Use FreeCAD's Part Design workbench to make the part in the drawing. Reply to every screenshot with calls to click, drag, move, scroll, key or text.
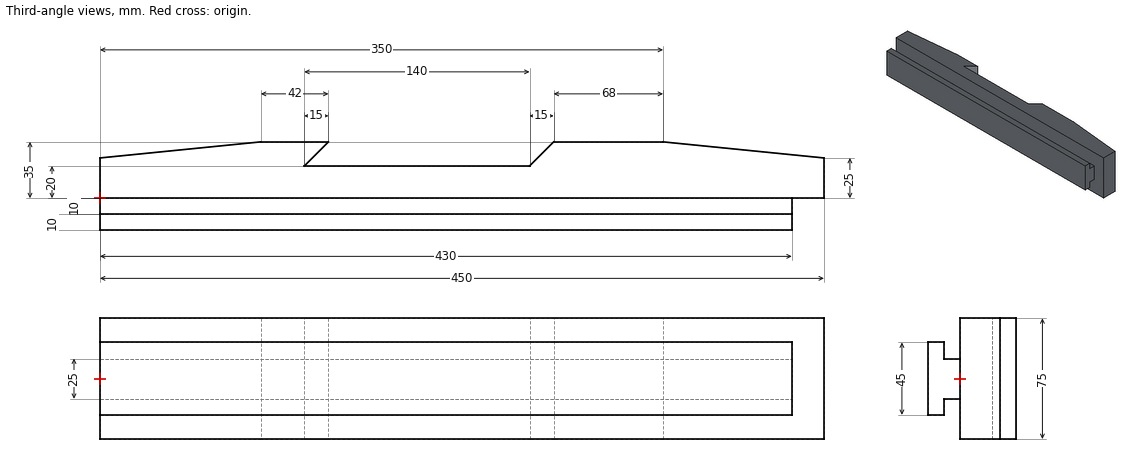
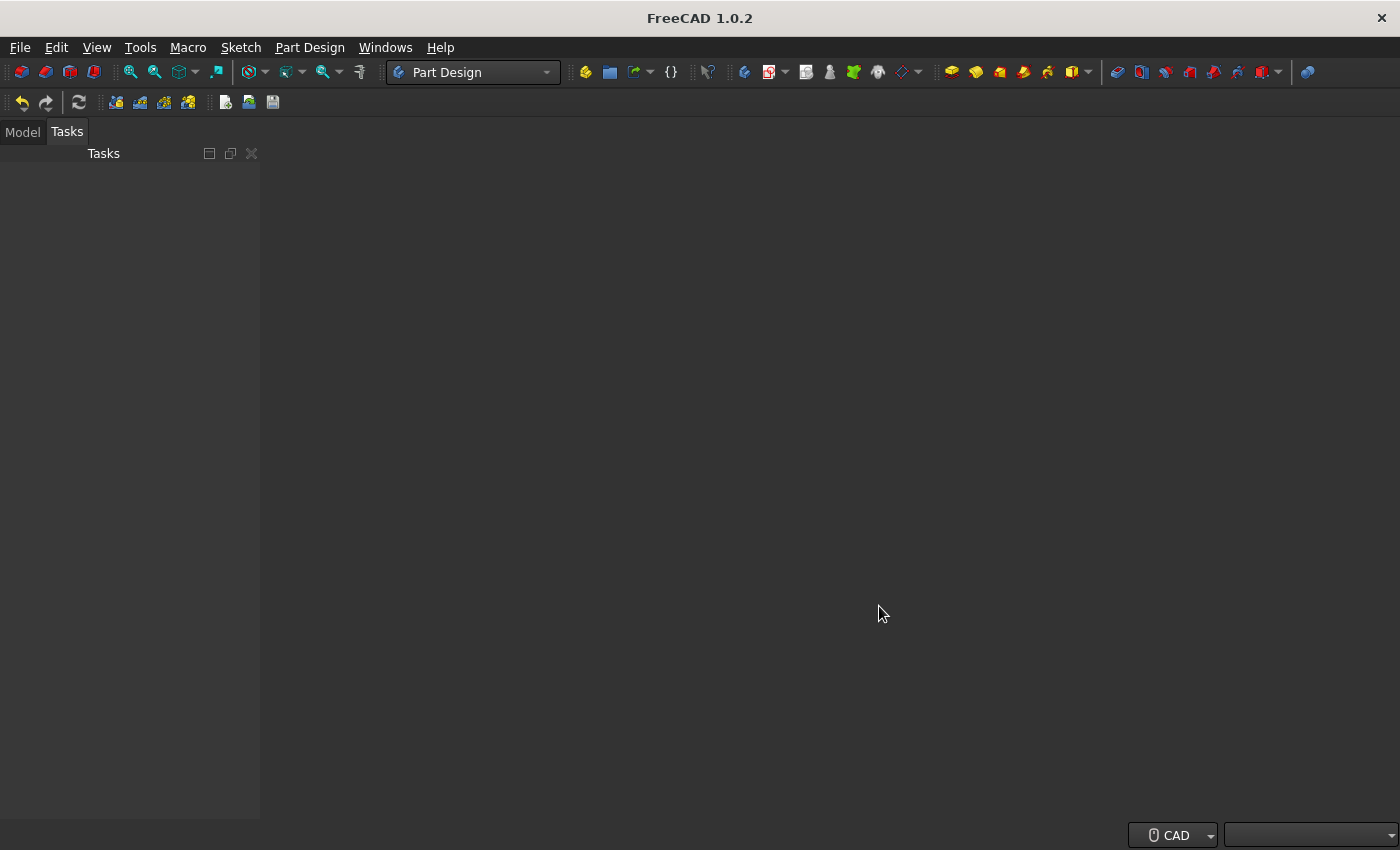
click(226, 102)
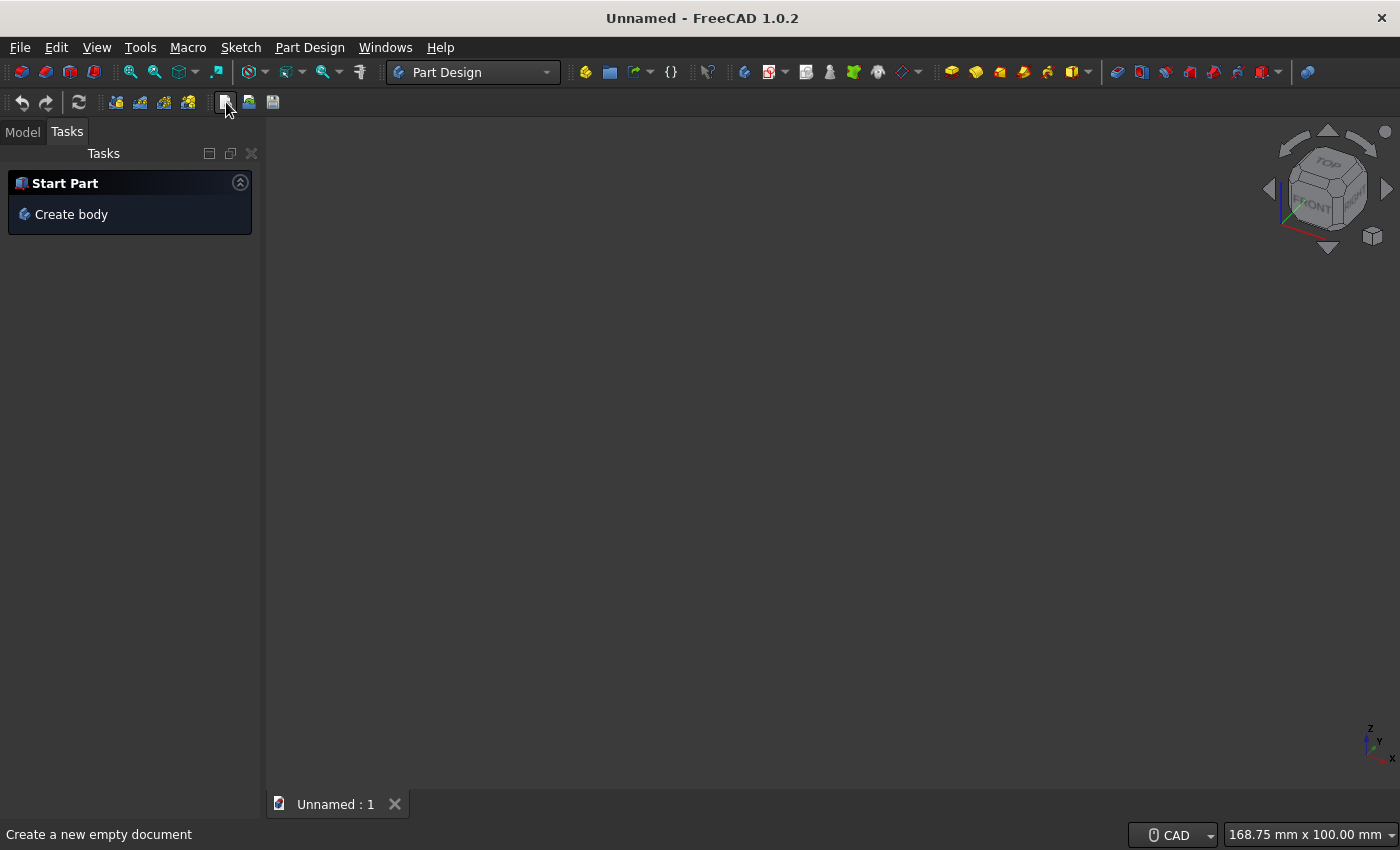
click(770, 72)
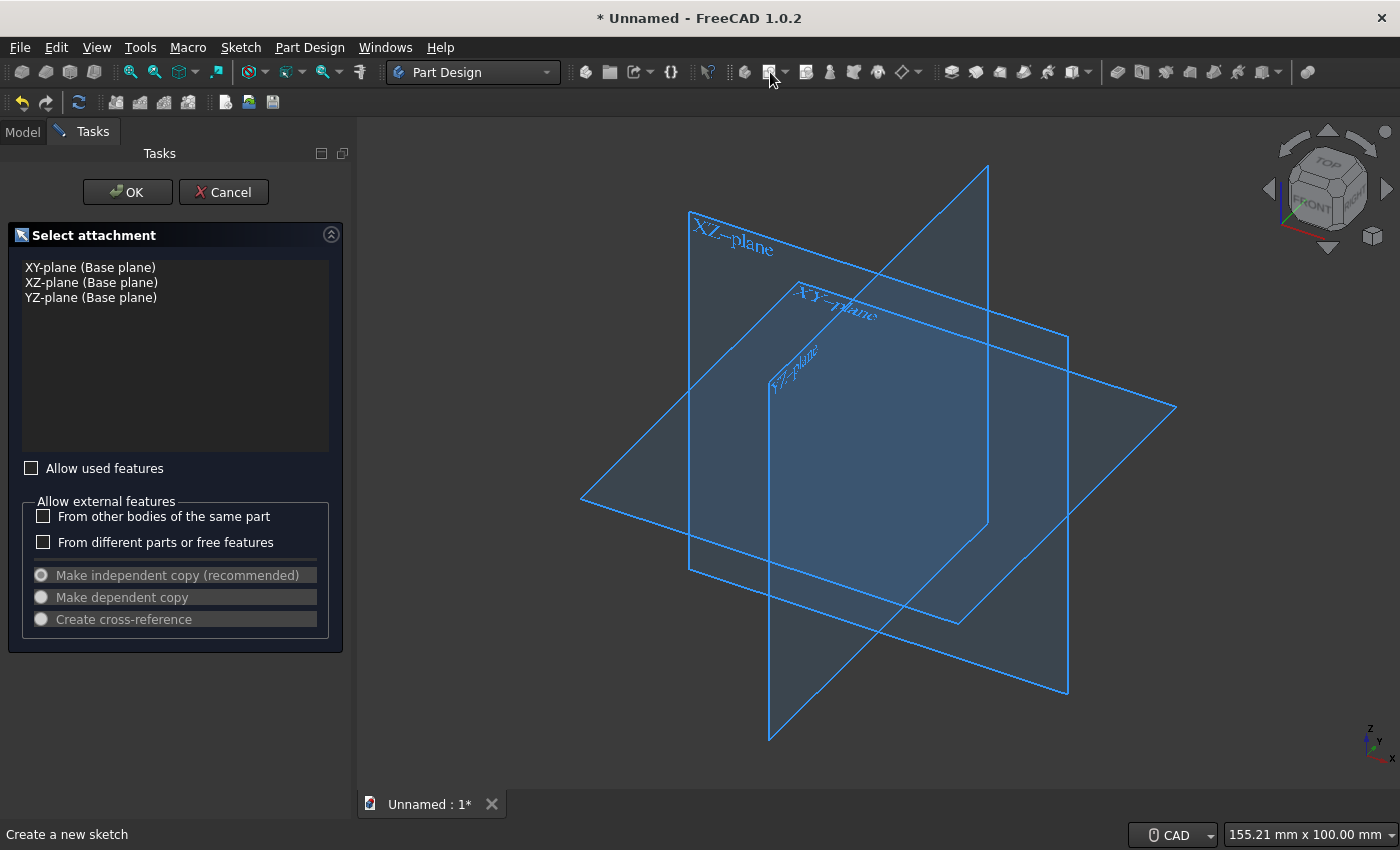
click(82, 268)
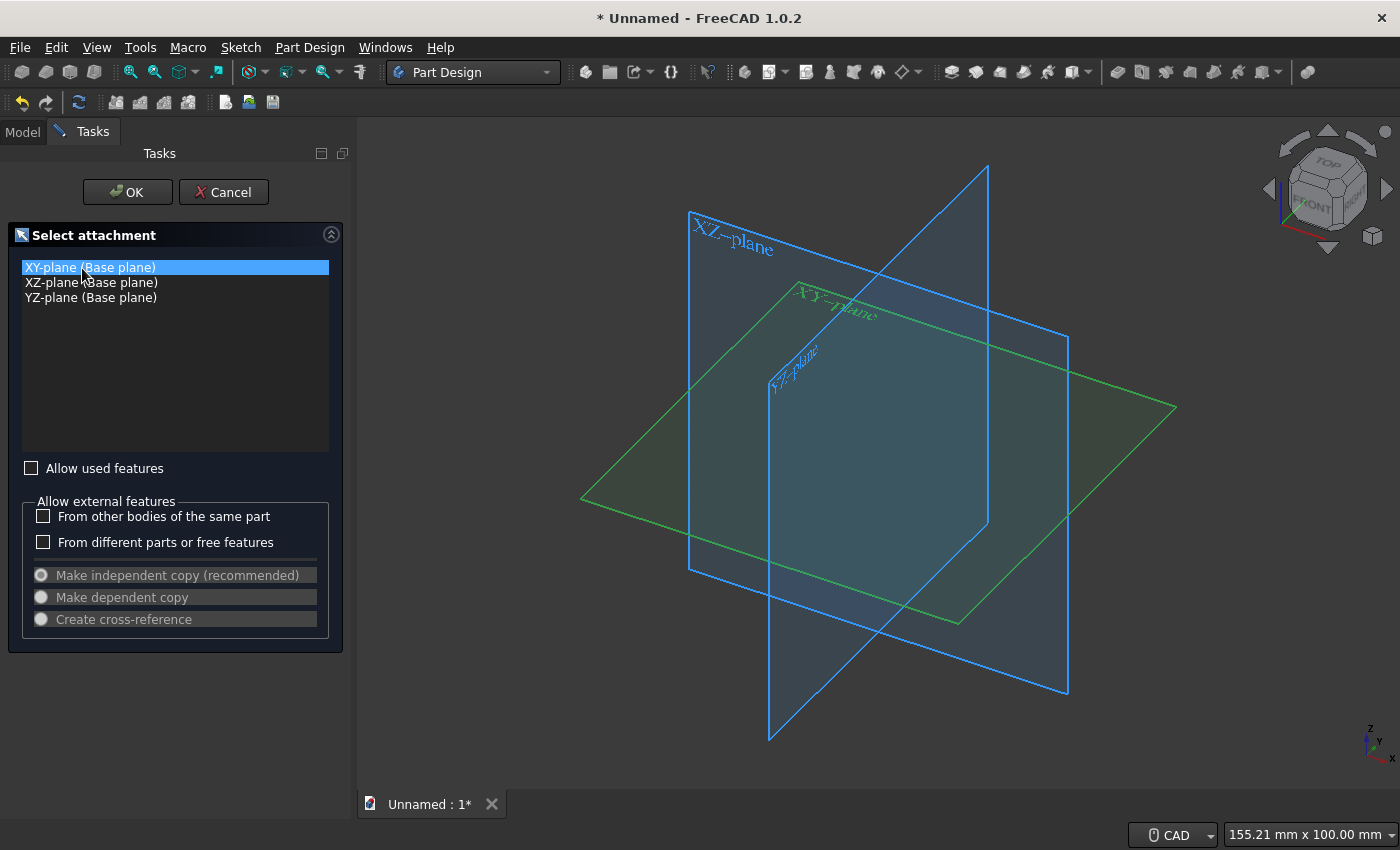
click(128, 192)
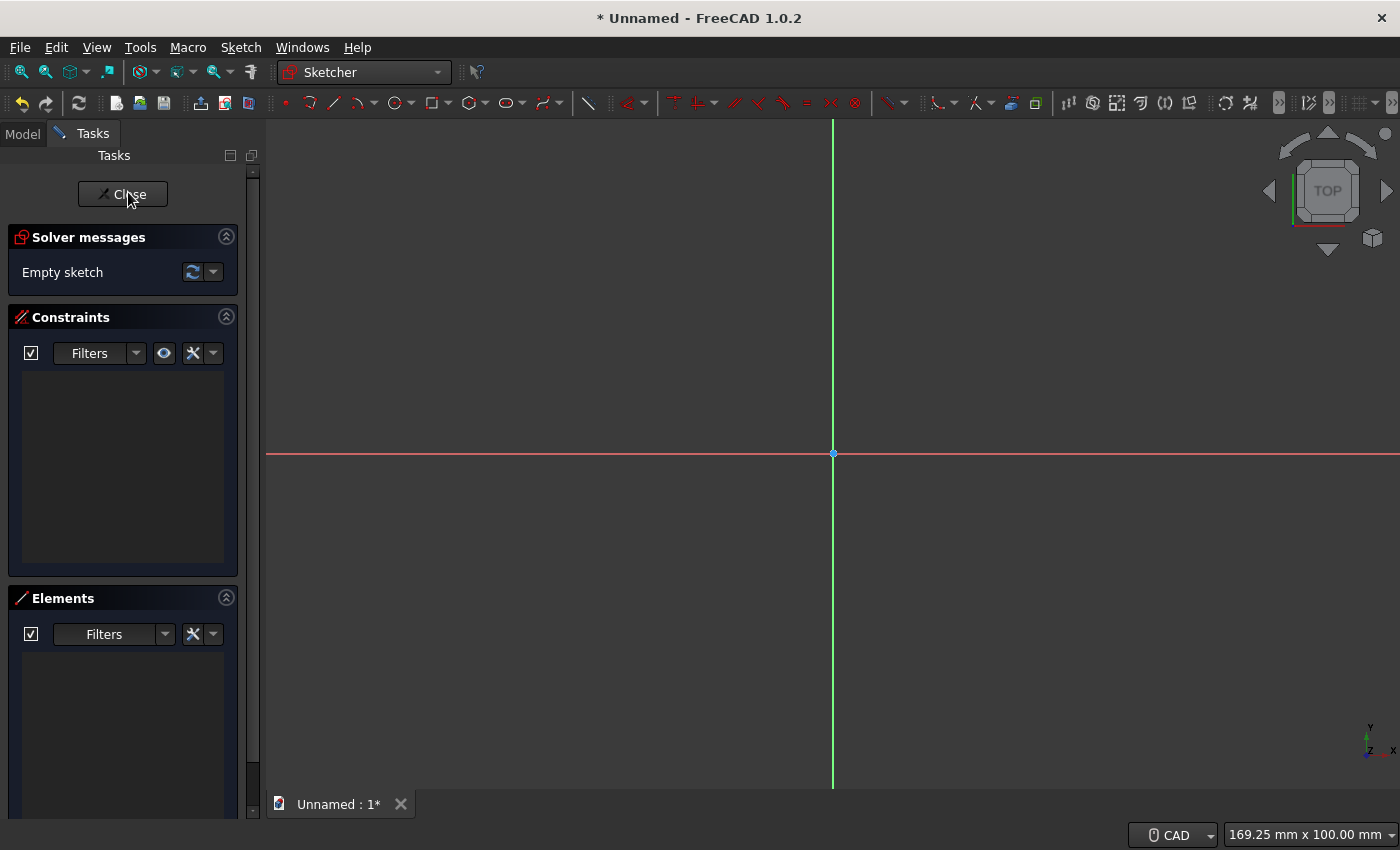
scroll(366, 484, down, 8)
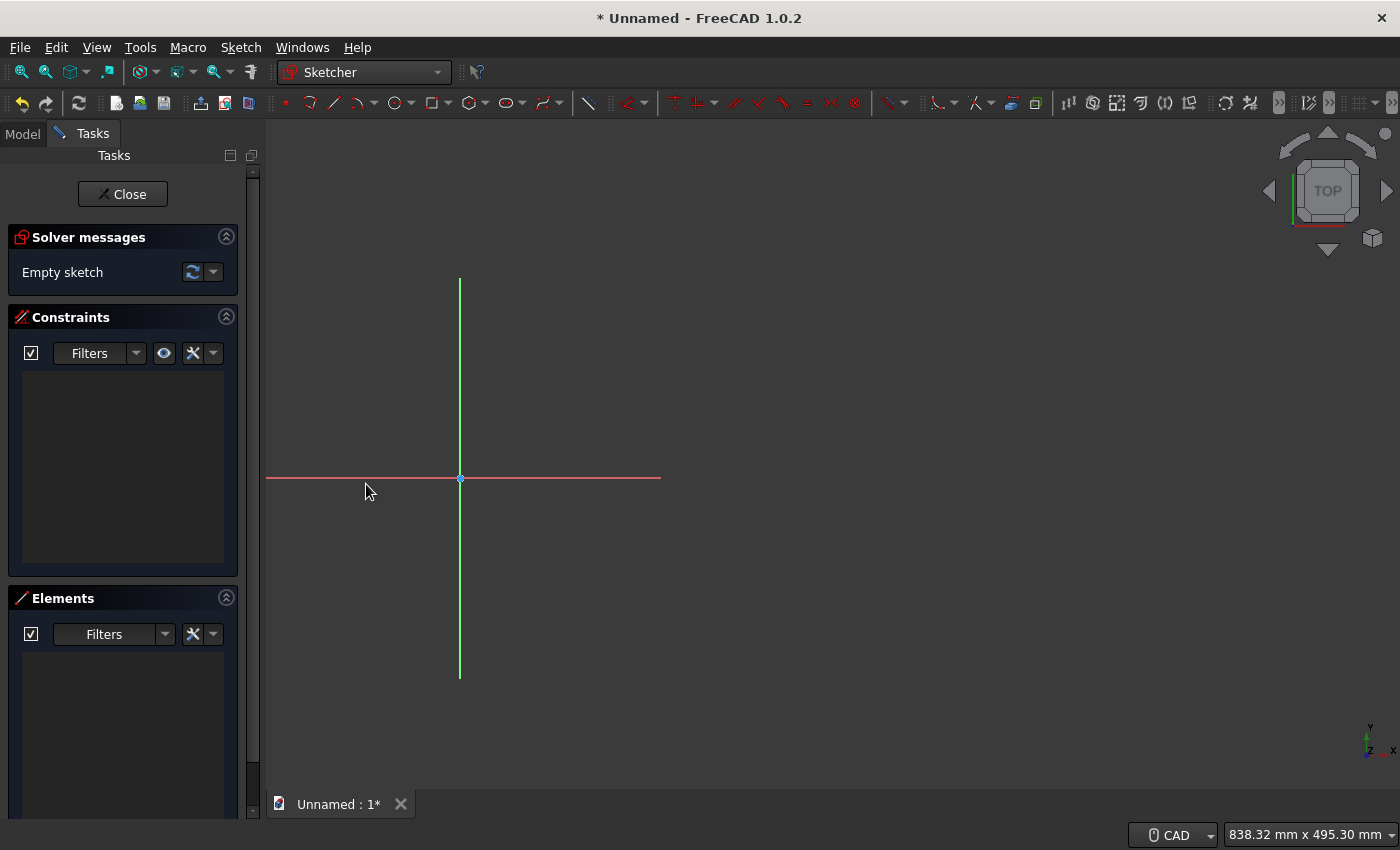
click(310, 104)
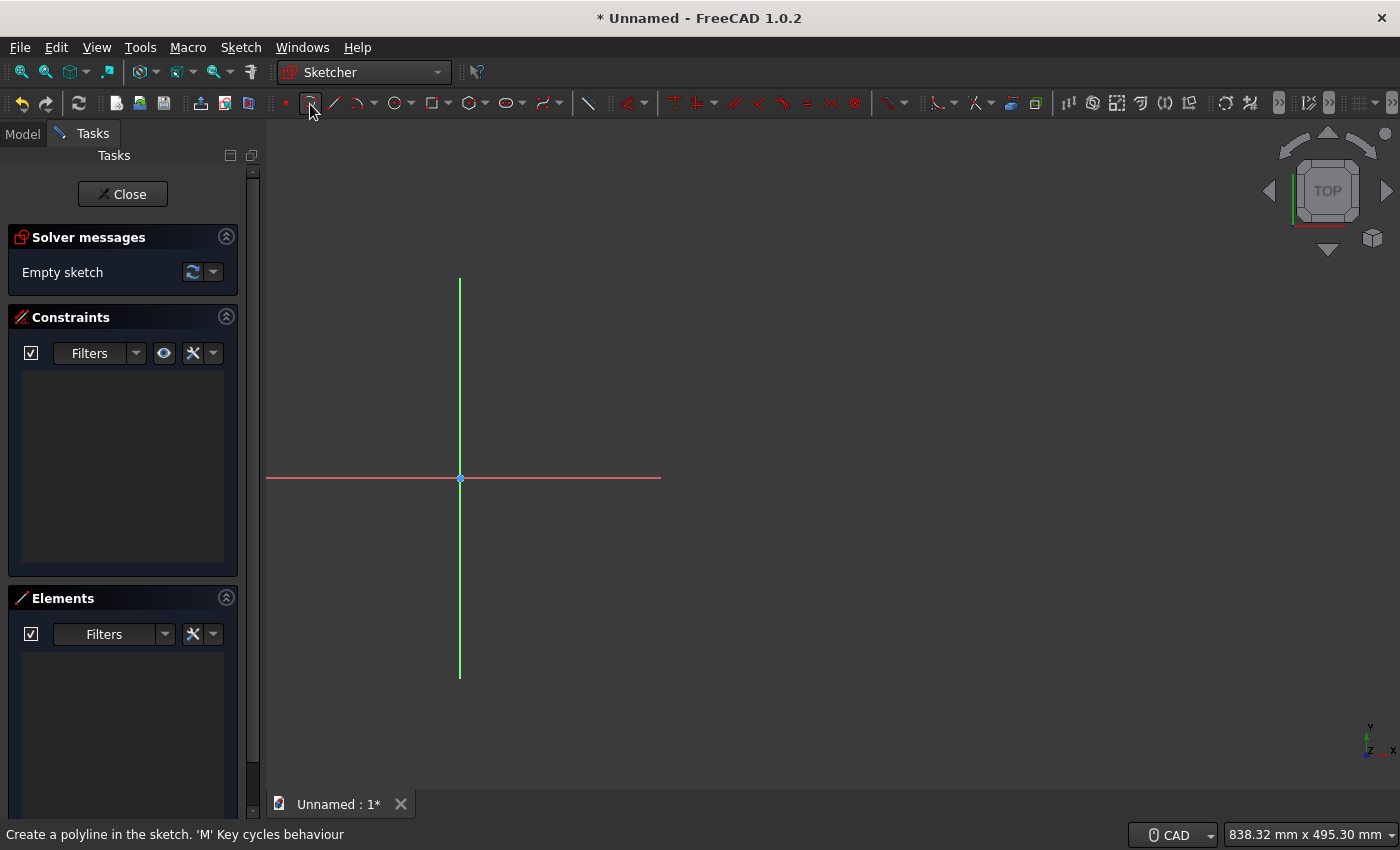
click(460, 478)
click(1069, 469)
click(1069, 445)
click(934, 431)
click(842, 431)
click(822, 451)
click(632, 451)
click(652, 431)
click(596, 431)
click(469, 445)
click(460, 478)
key(Escape)
key(Escape)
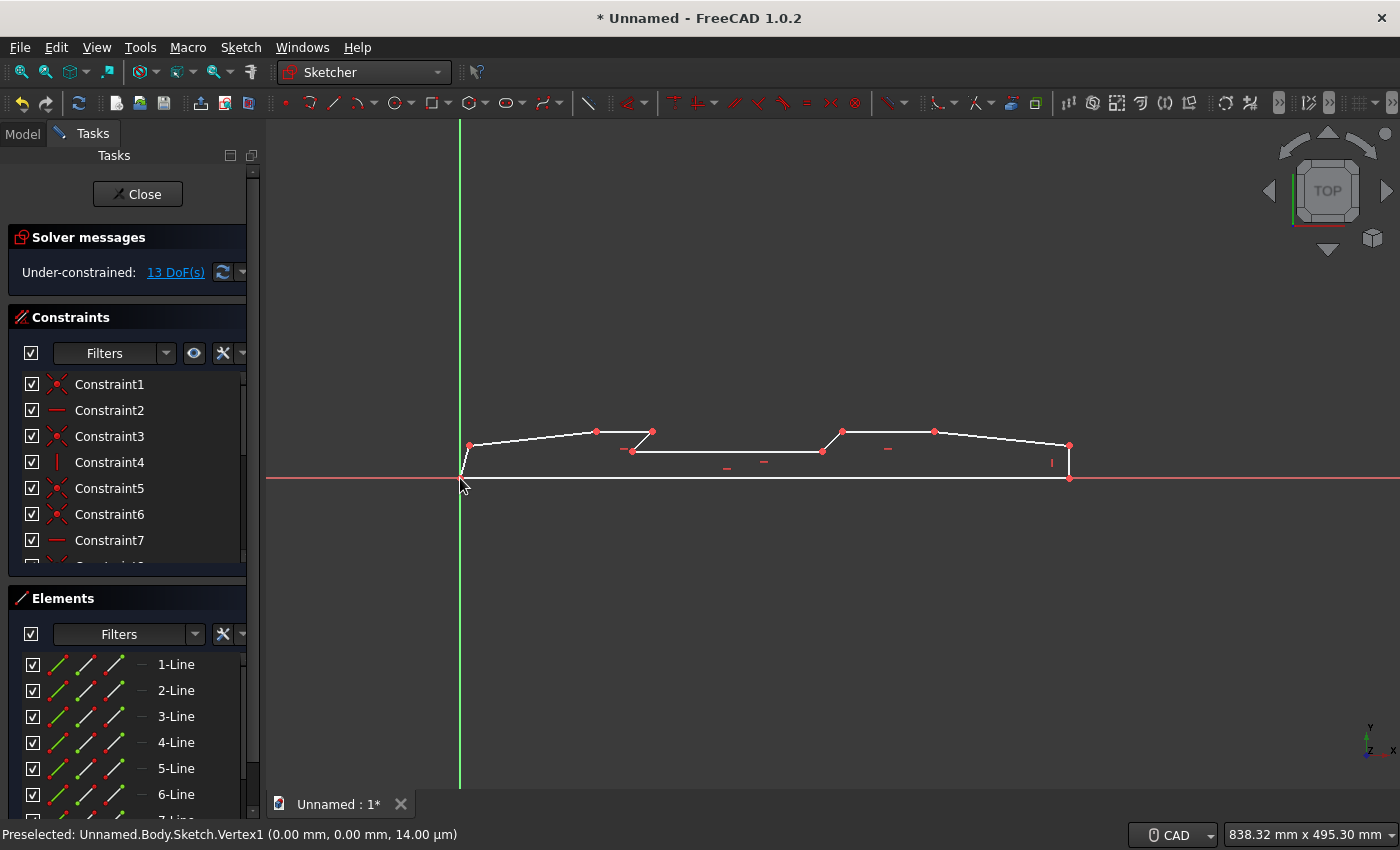
scroll(463, 469, up, 2)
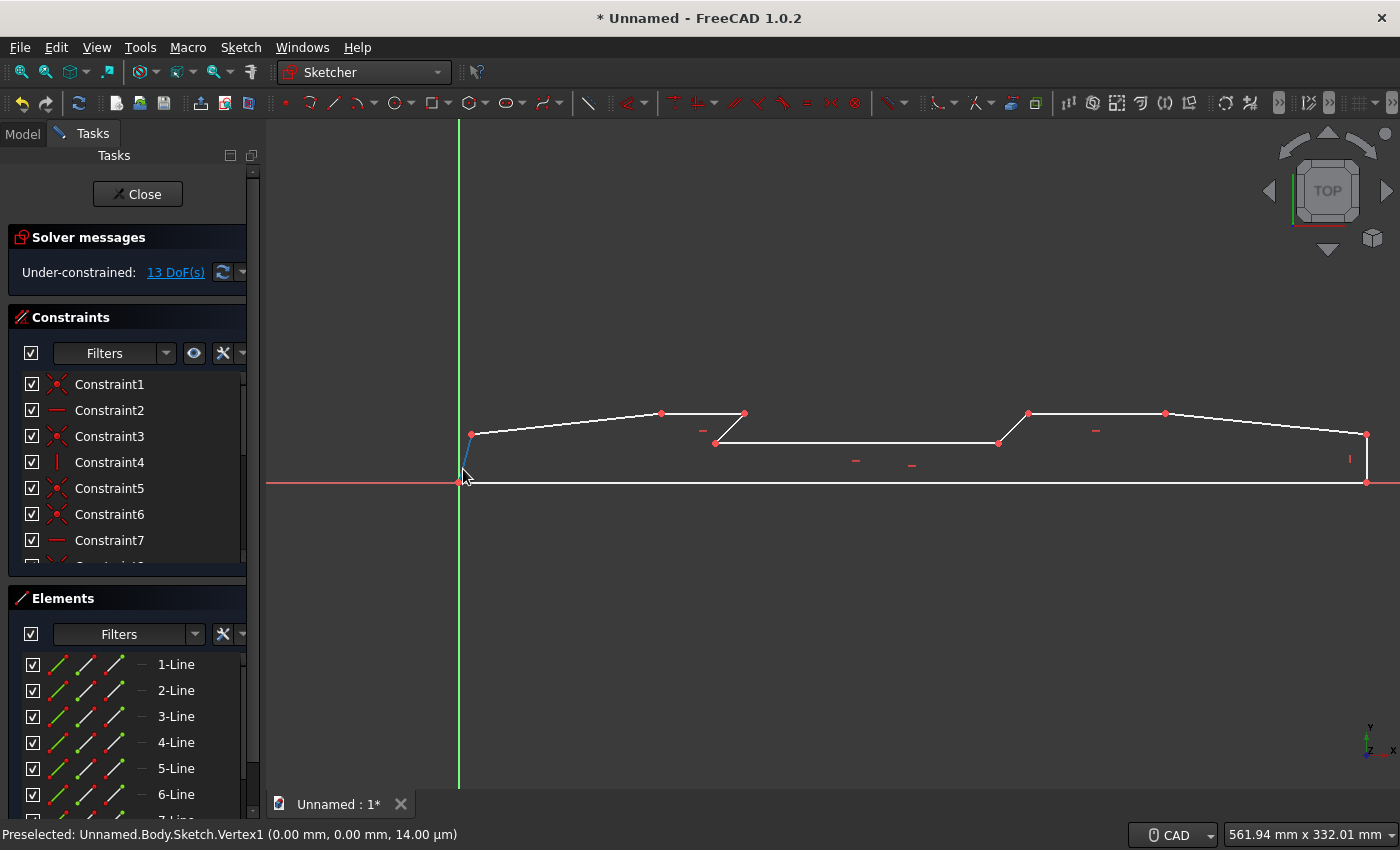
click(463, 468)